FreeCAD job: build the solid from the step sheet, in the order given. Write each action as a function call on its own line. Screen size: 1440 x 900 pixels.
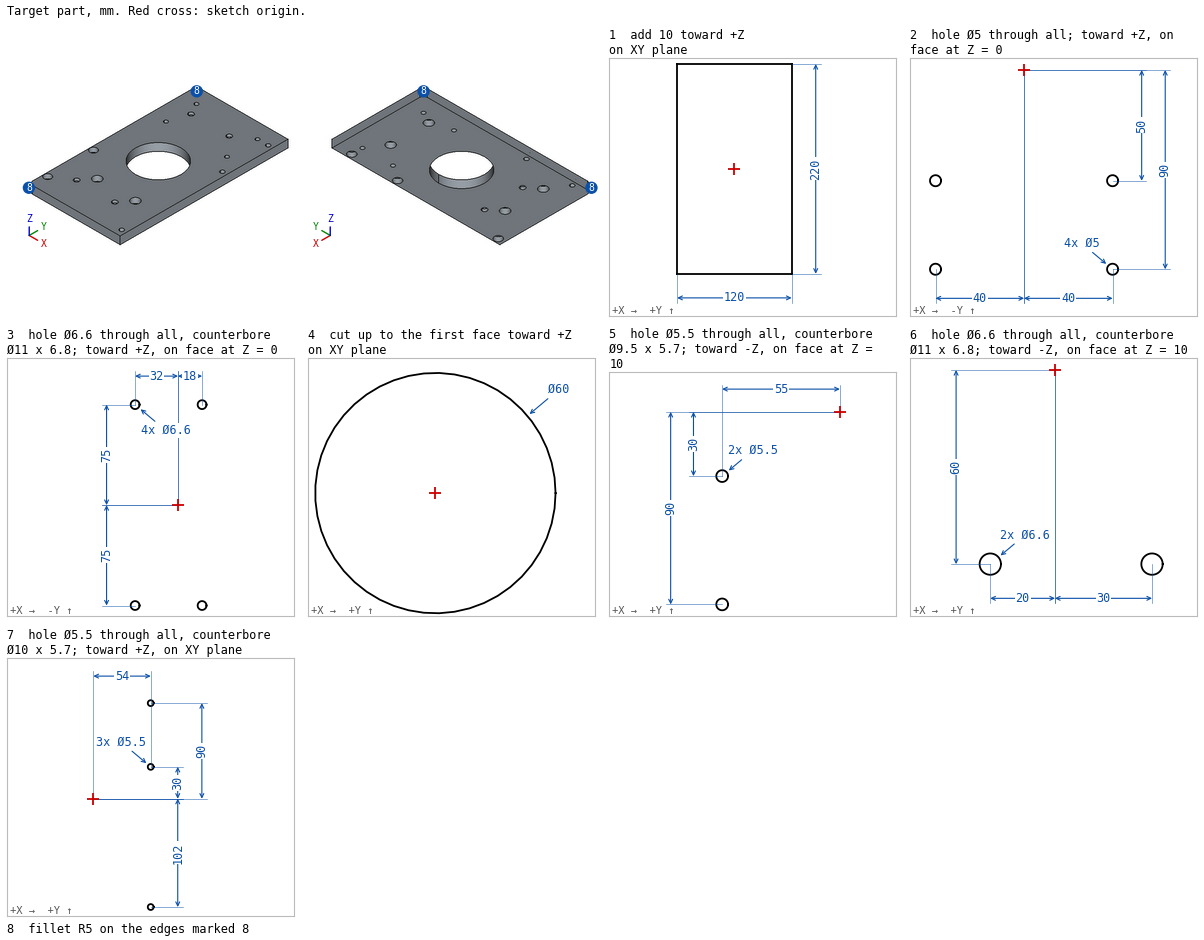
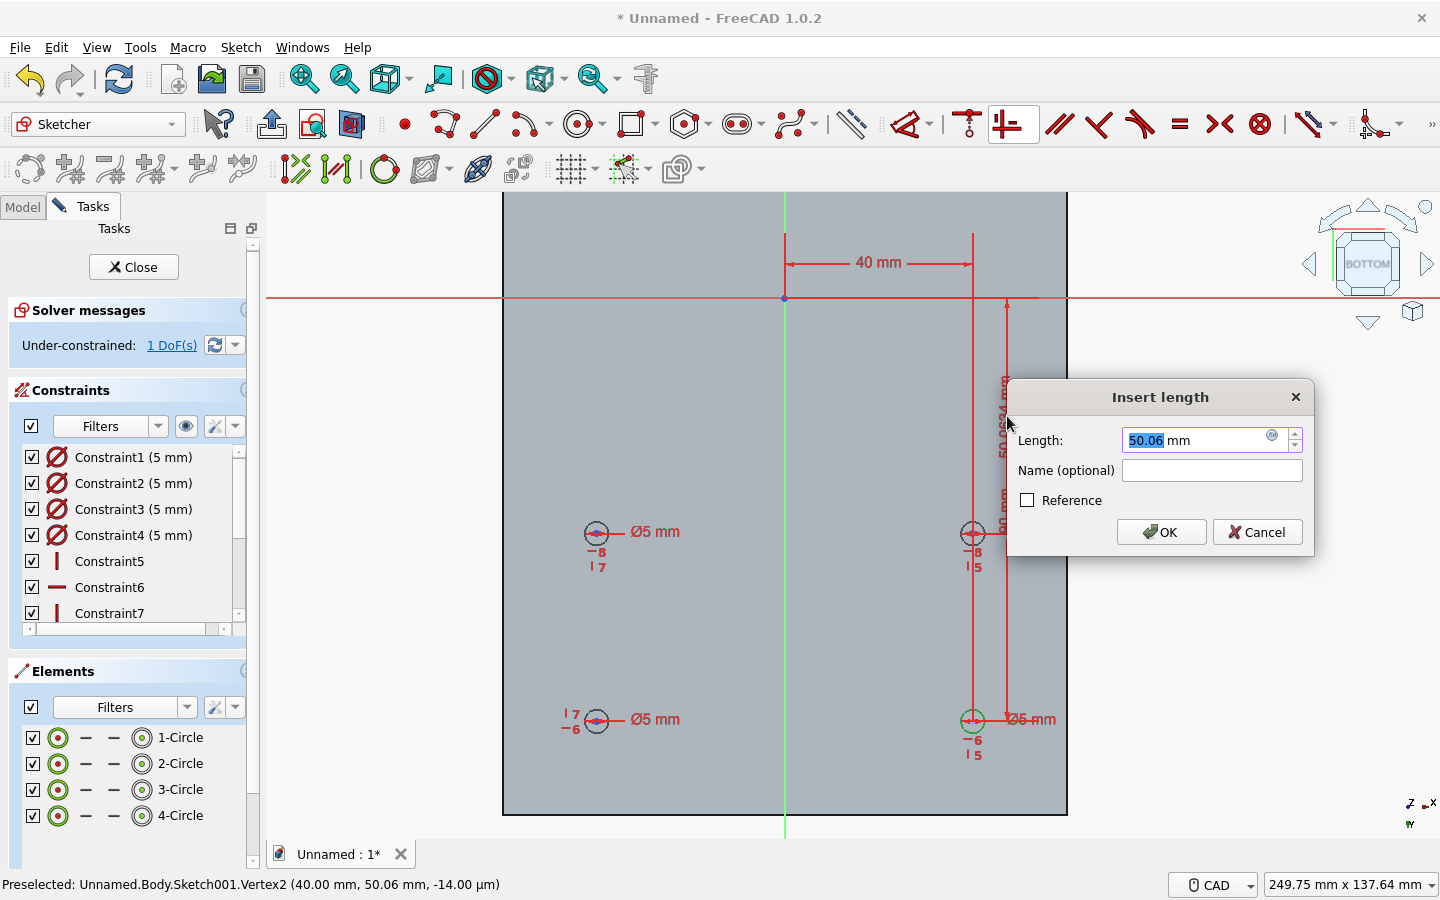
text(50)
key(Return)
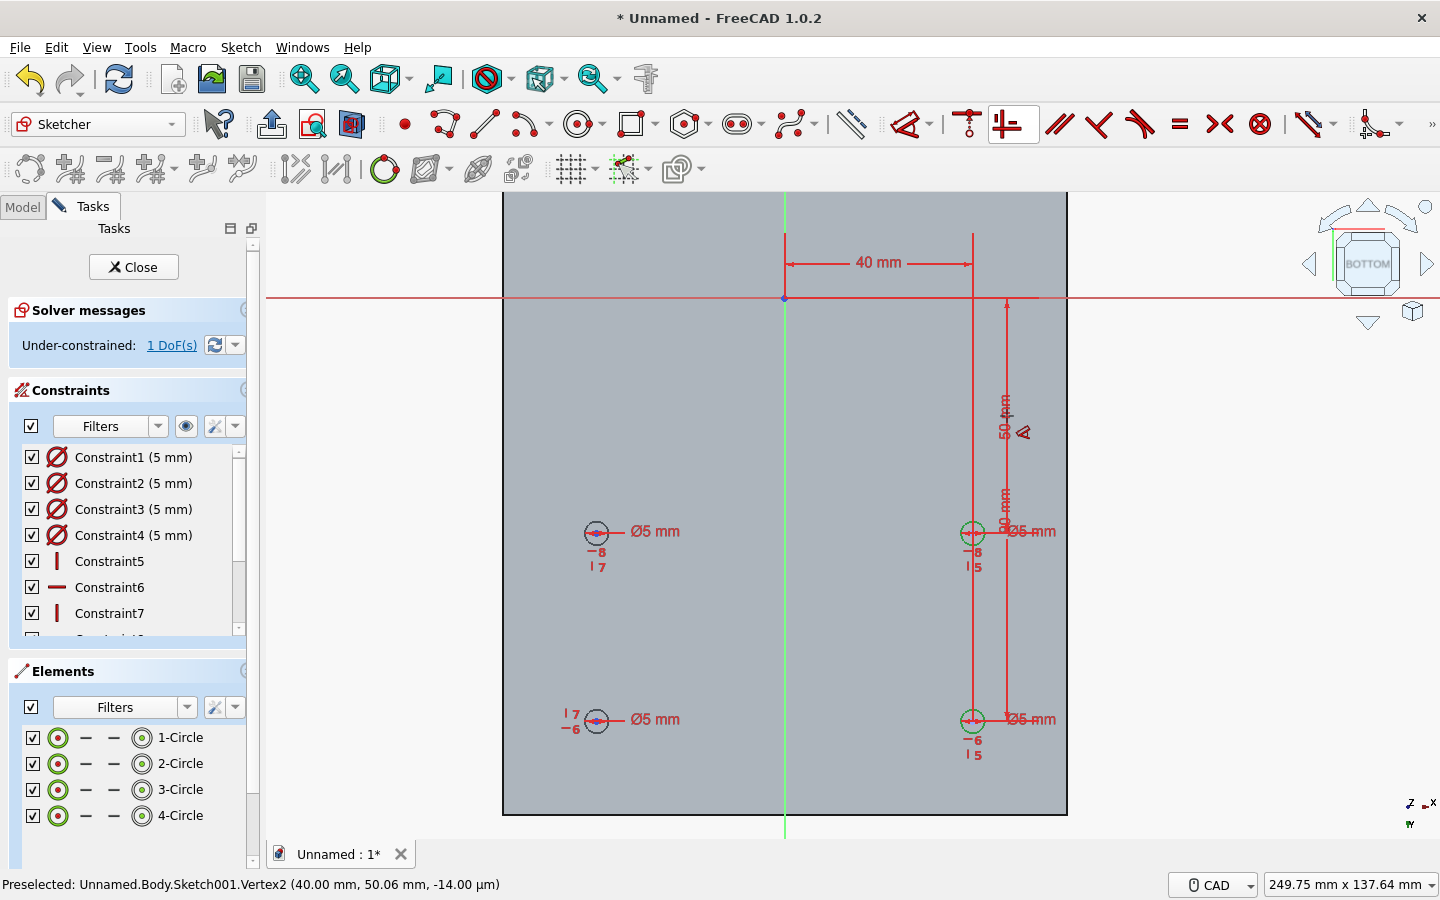
click(597, 721)
click(691, 264)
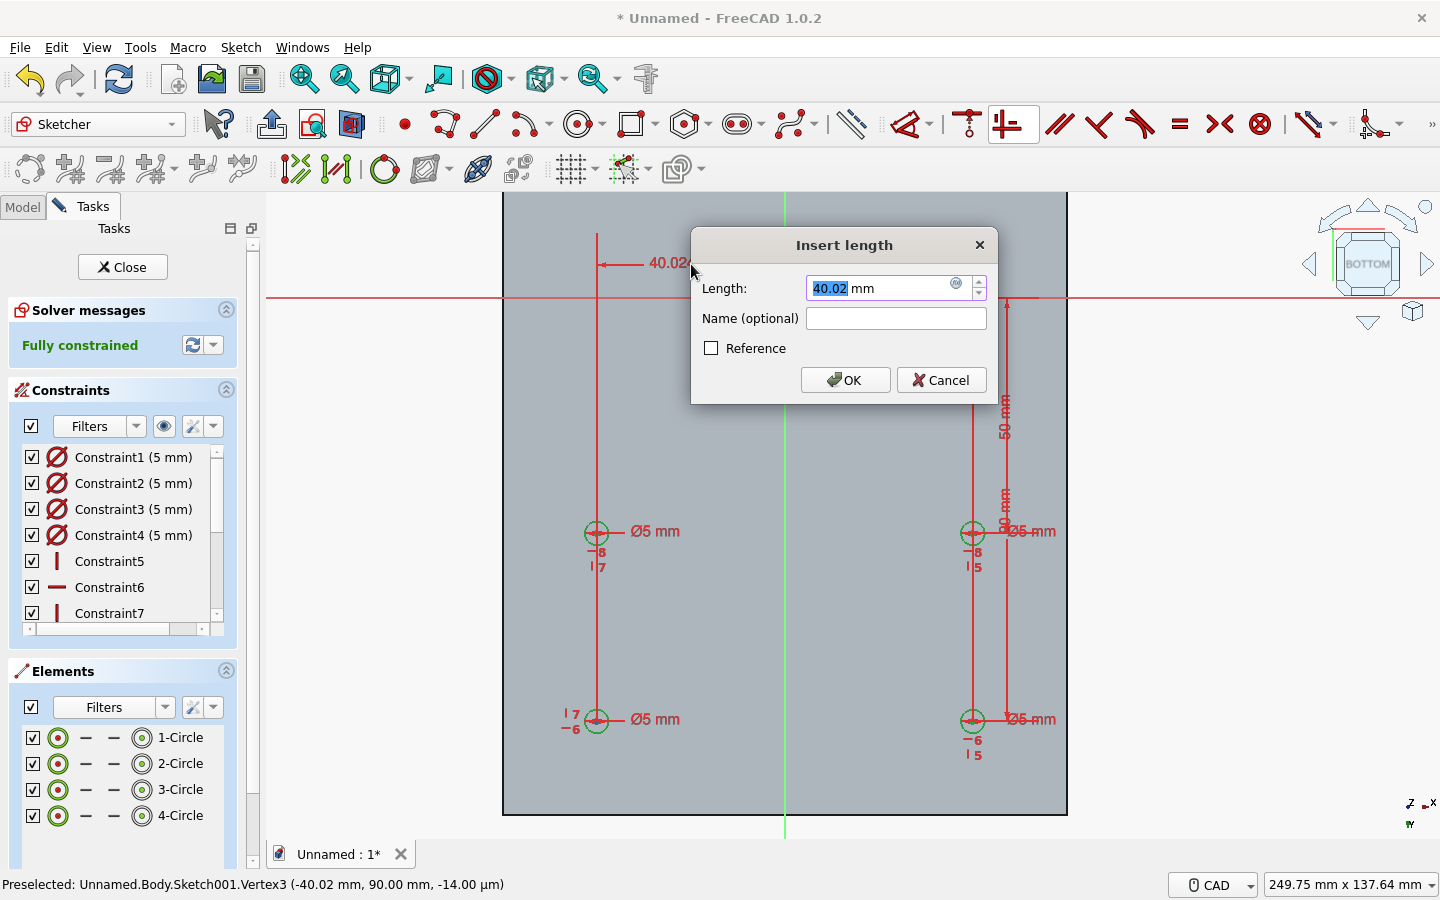
text(40)
key(Return)
key(Escape)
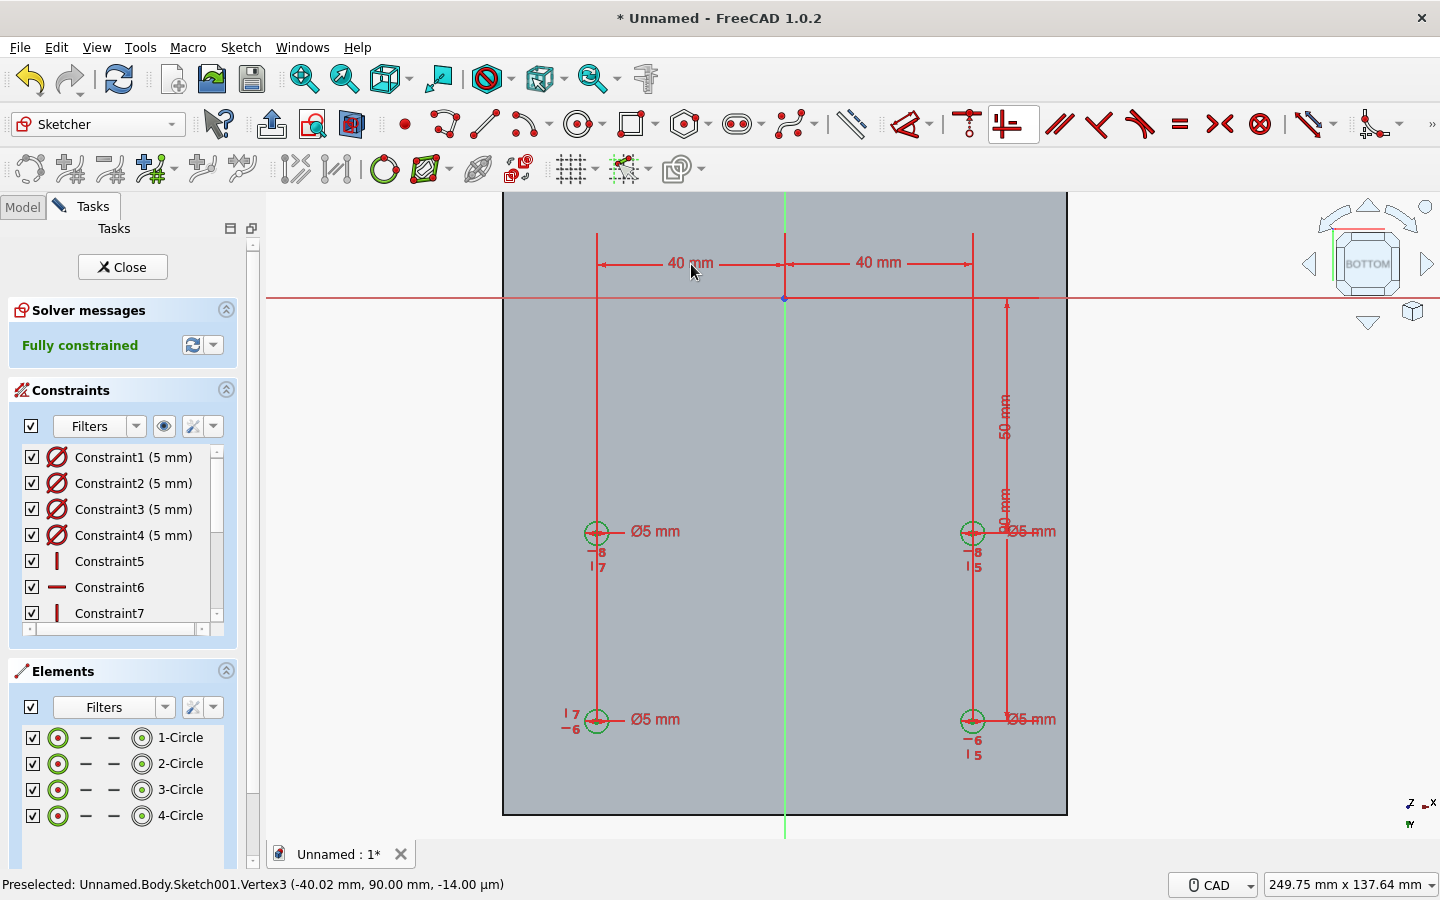
click(123, 267)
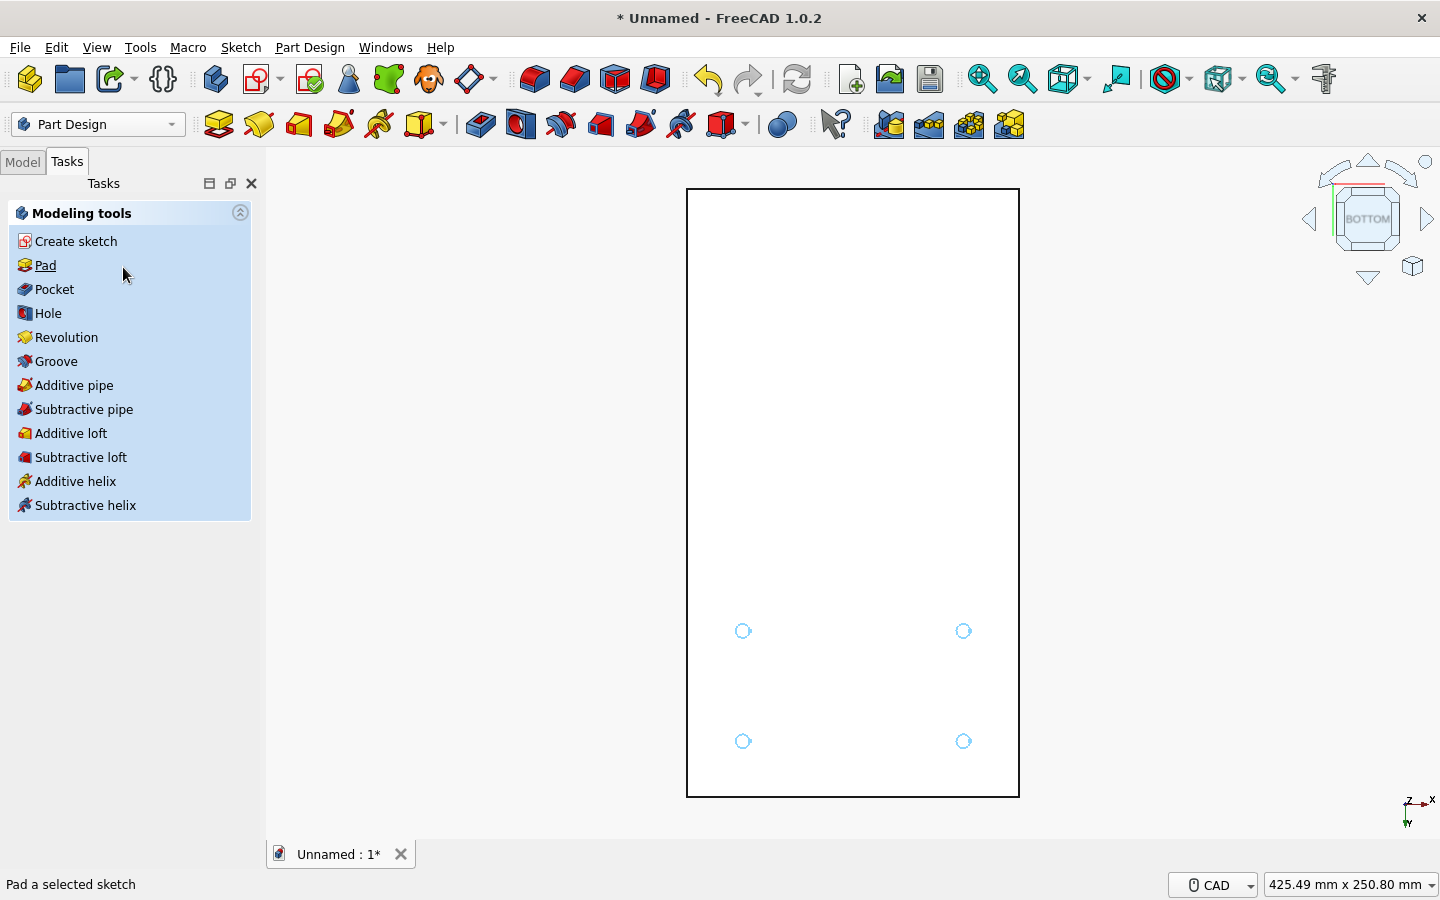
click(522, 124)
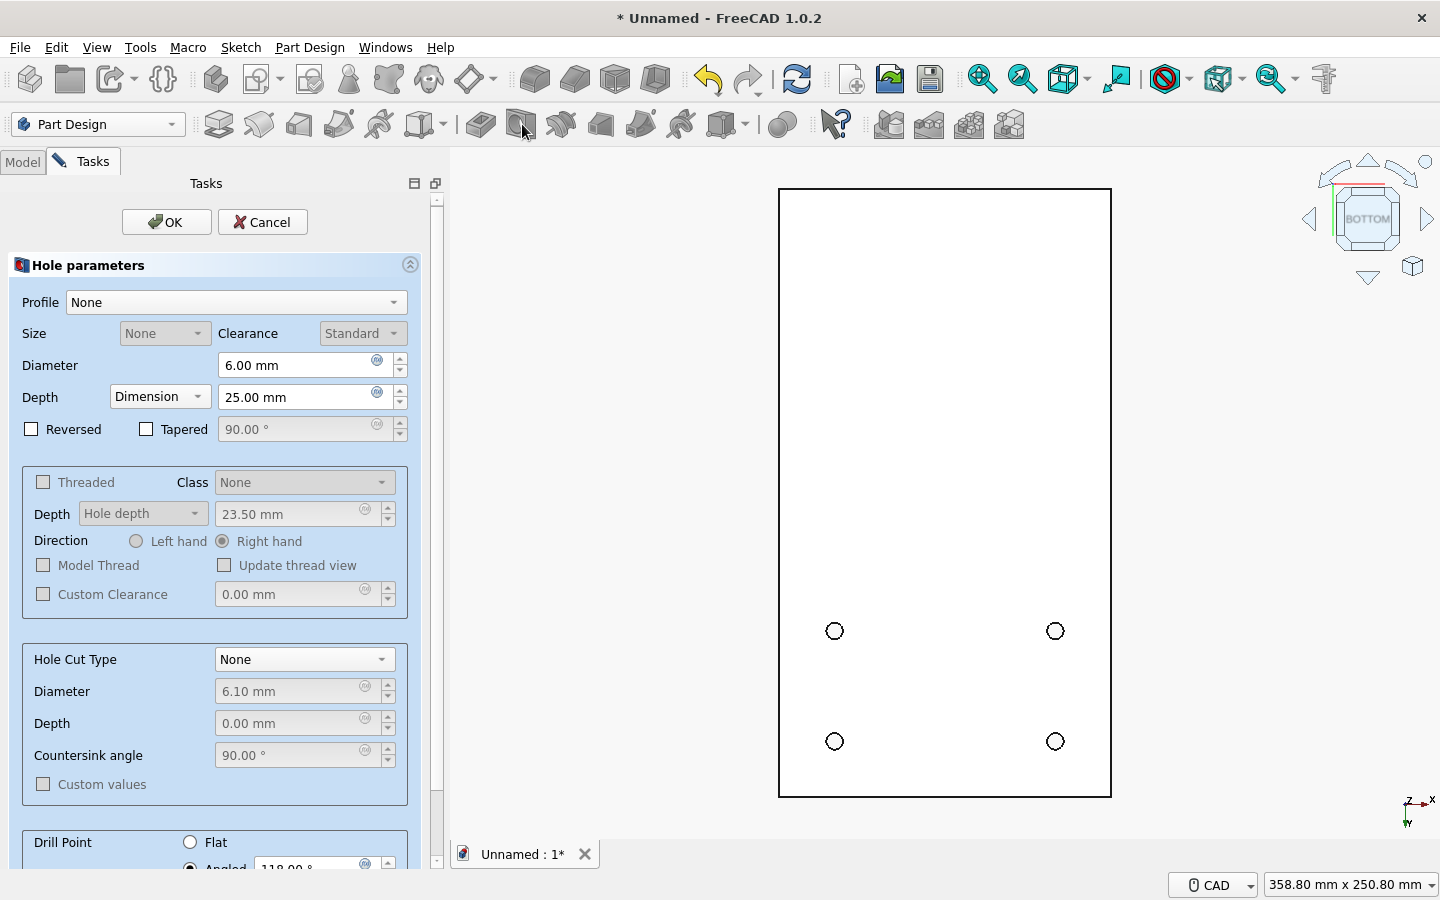
triple_click(305, 365)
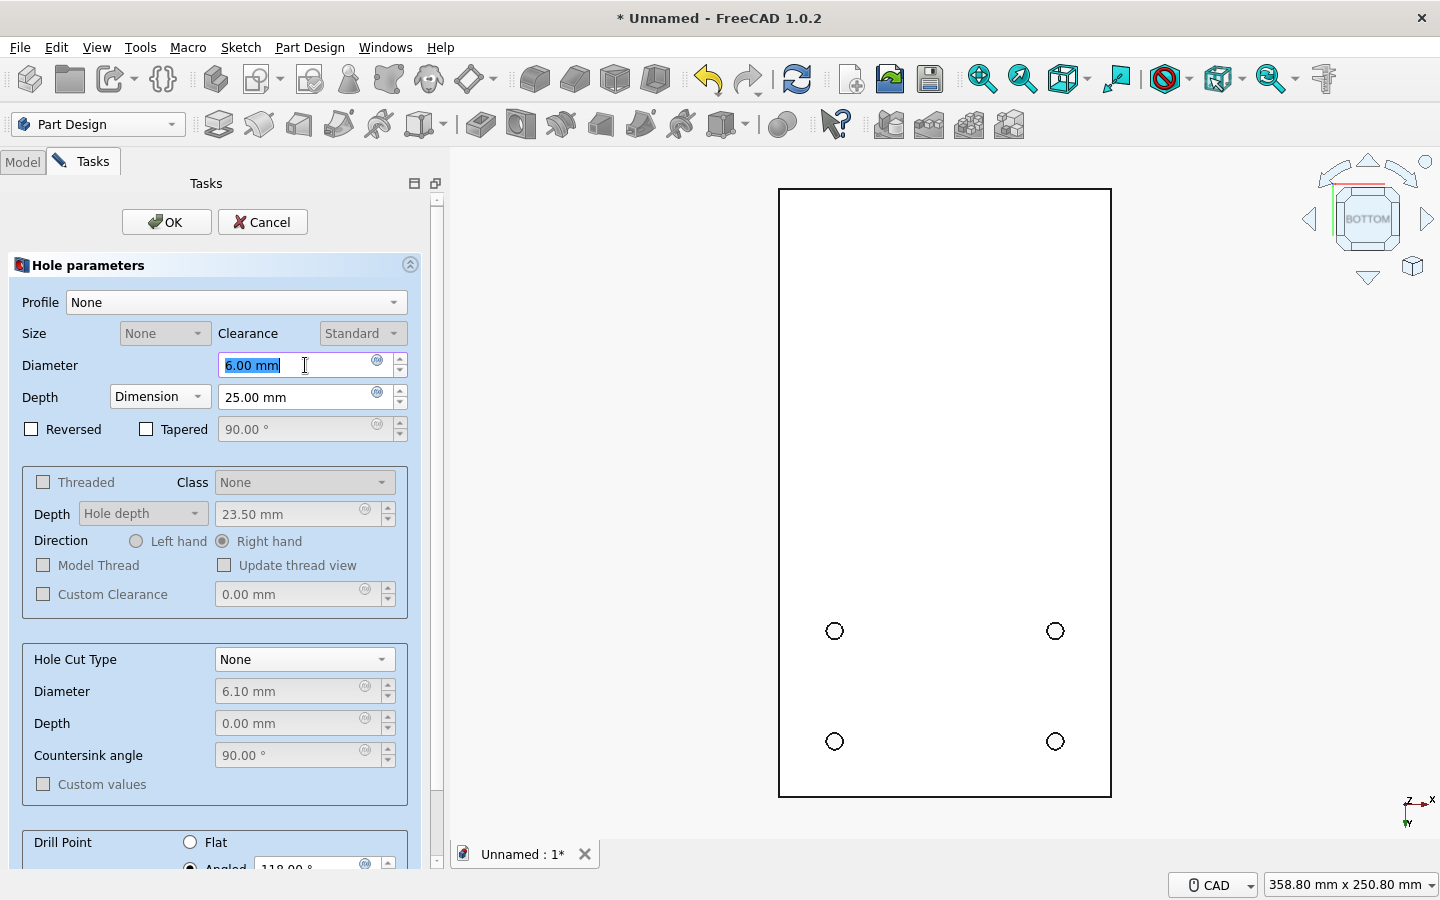
text(5)
key(Tab)